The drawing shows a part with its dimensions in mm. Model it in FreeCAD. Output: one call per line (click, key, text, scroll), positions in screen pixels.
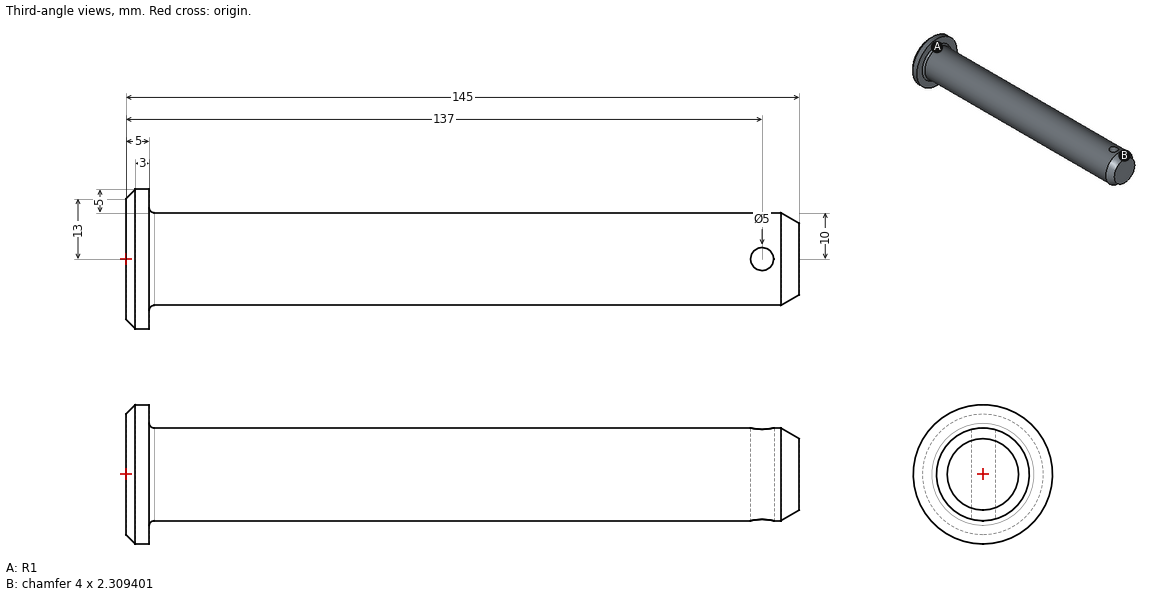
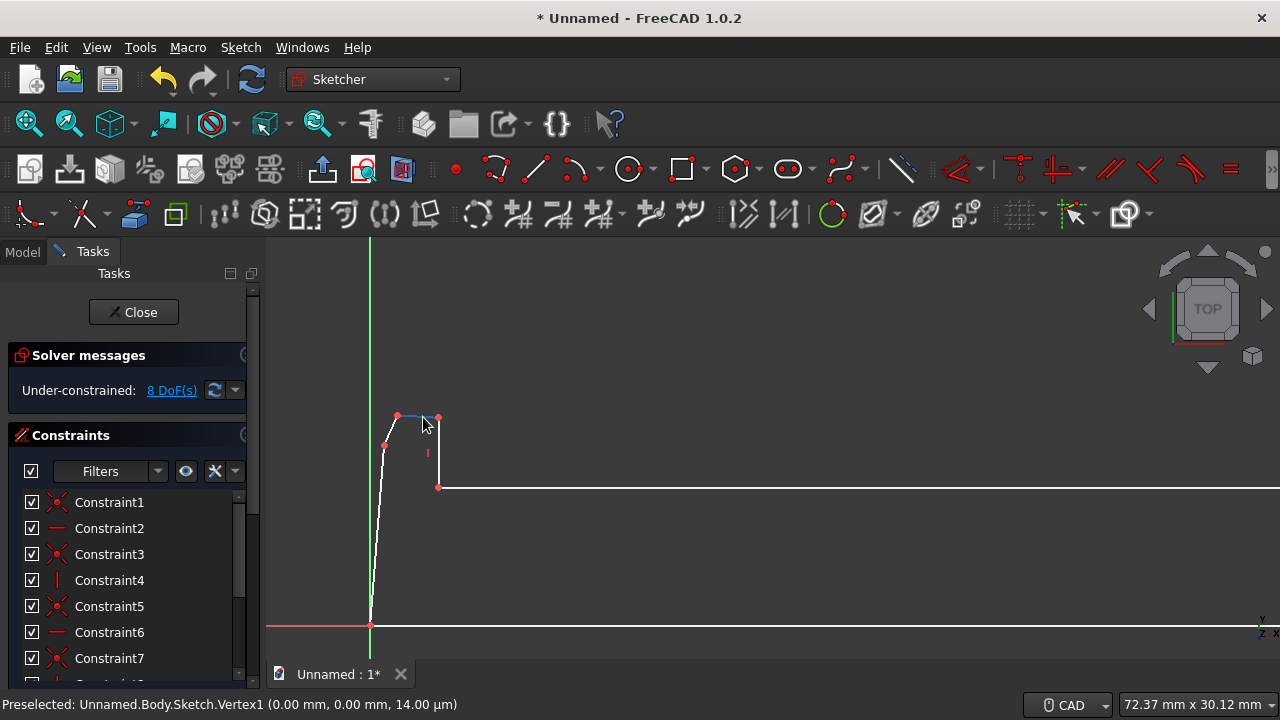
click(422, 417)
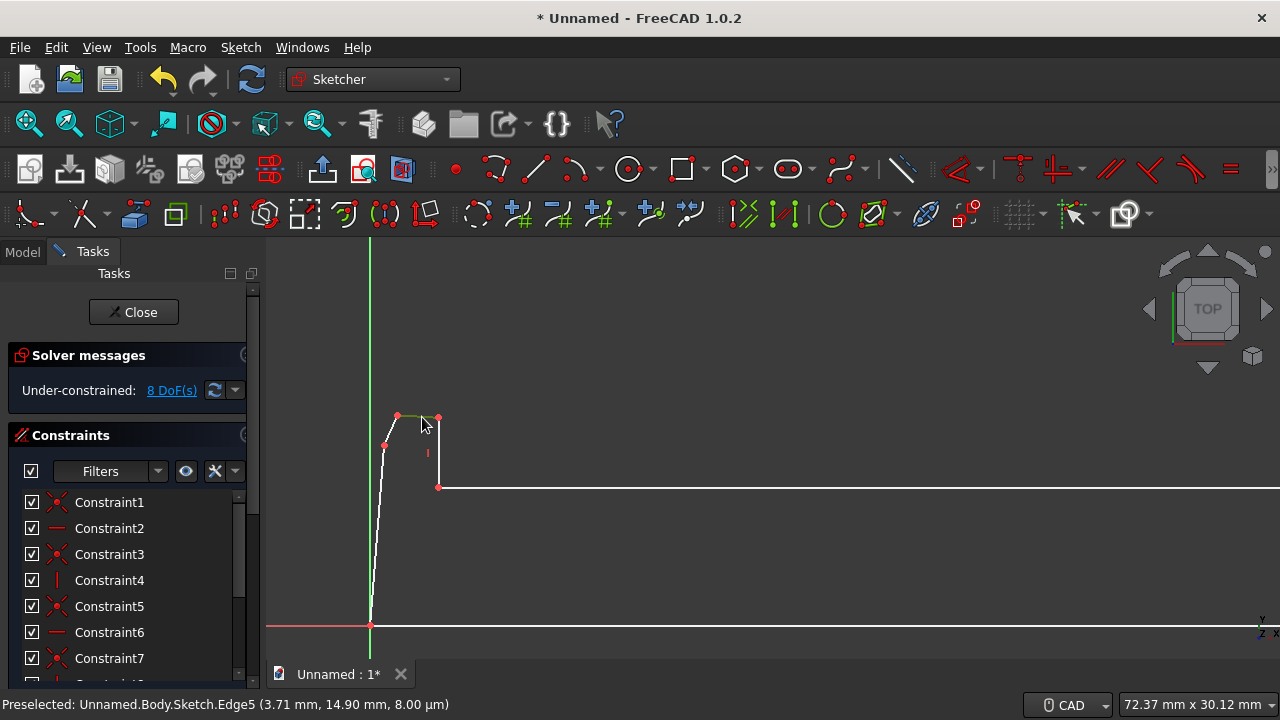
key(h)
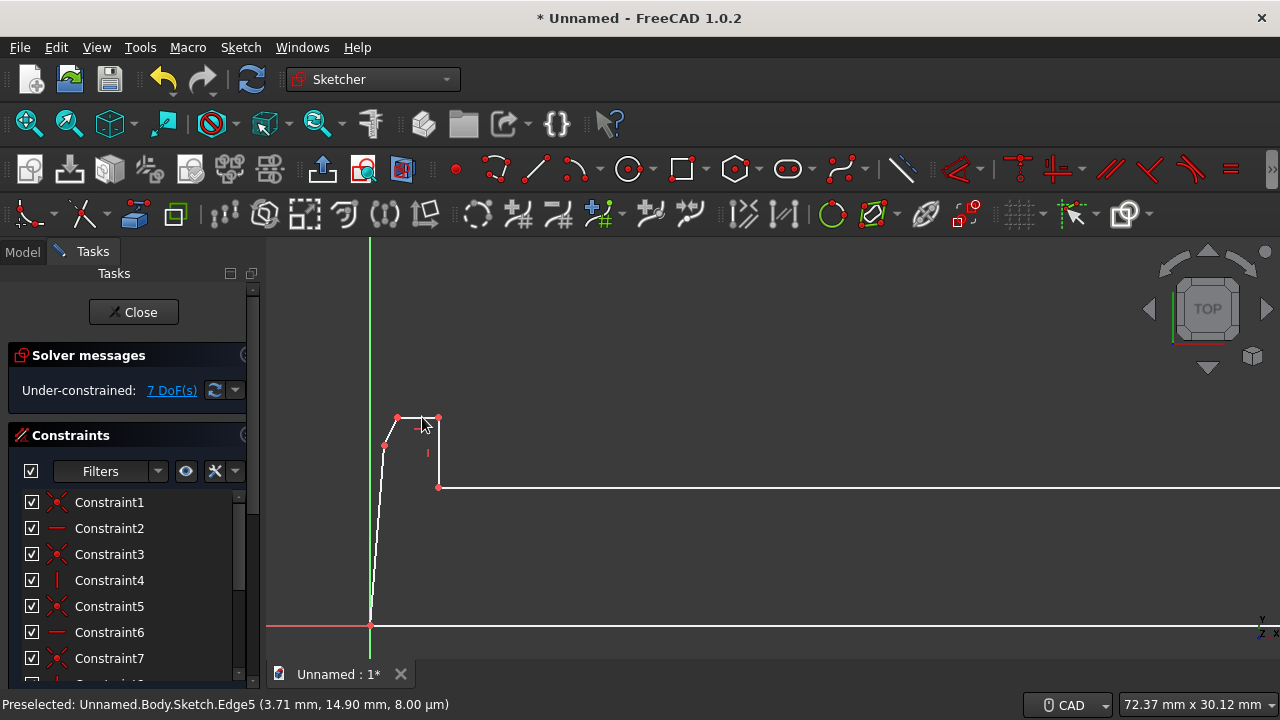
scroll(380, 499, up, 2)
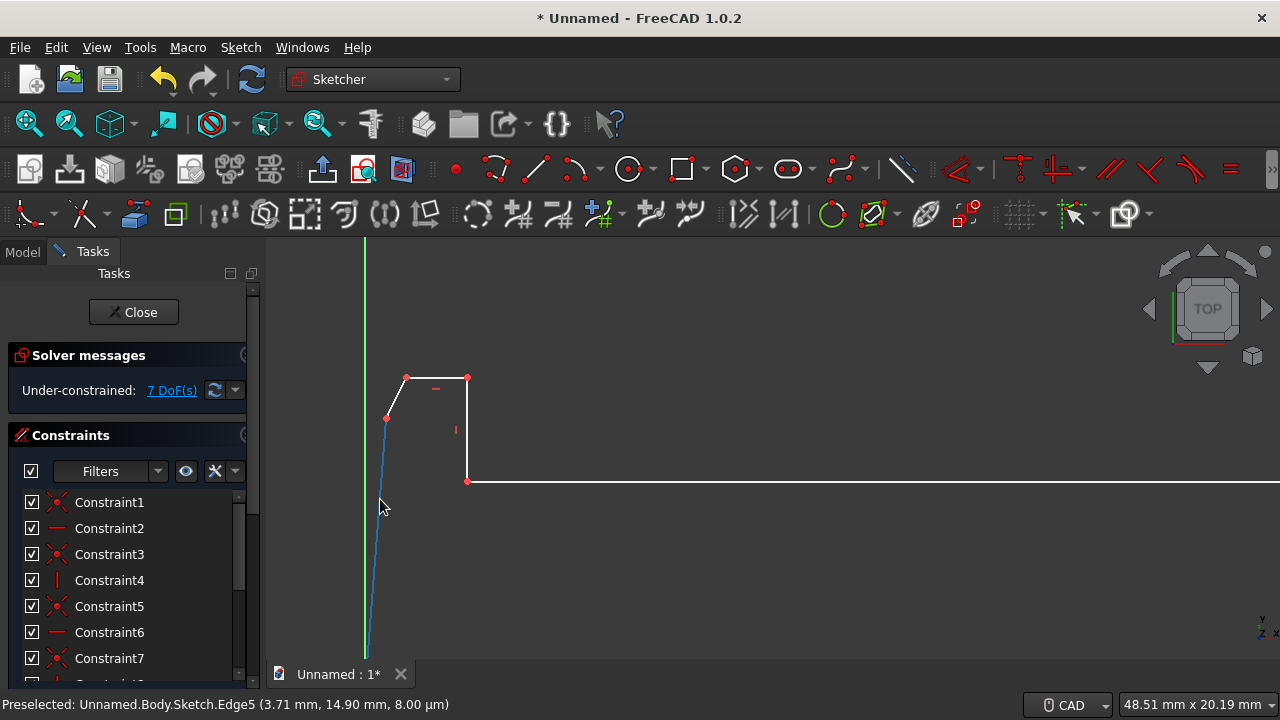
click(380, 499)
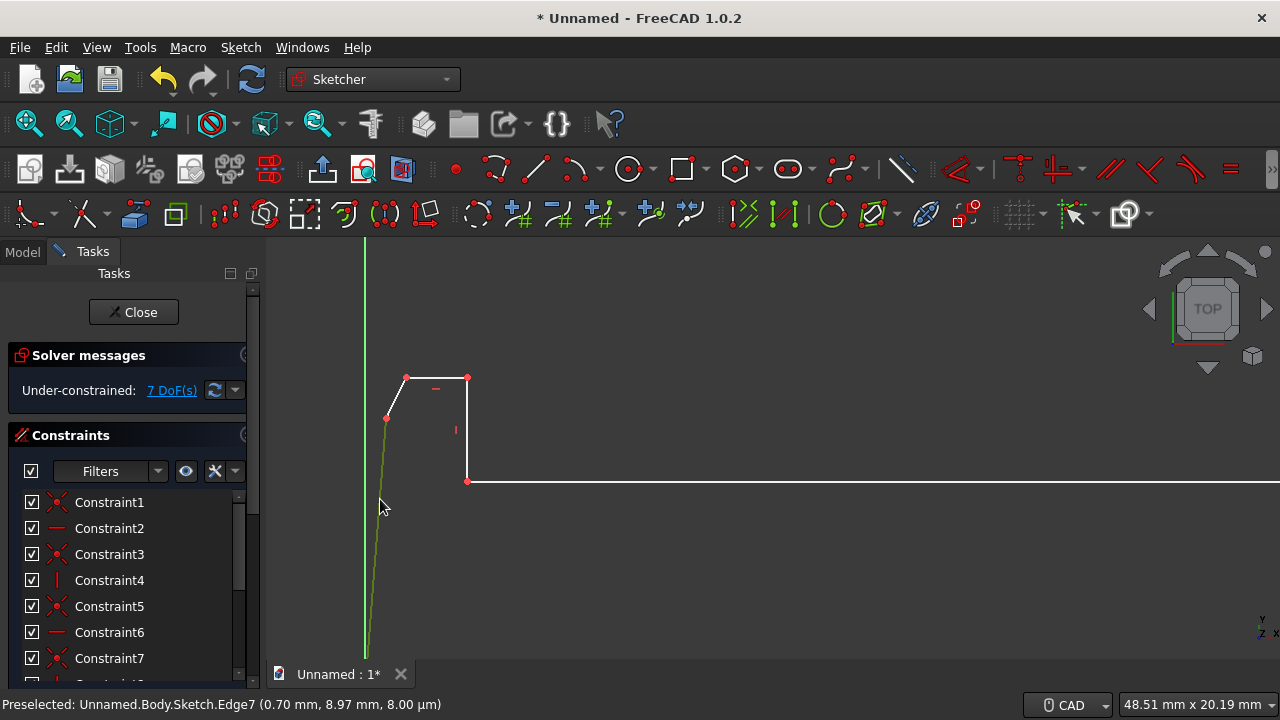
key(v)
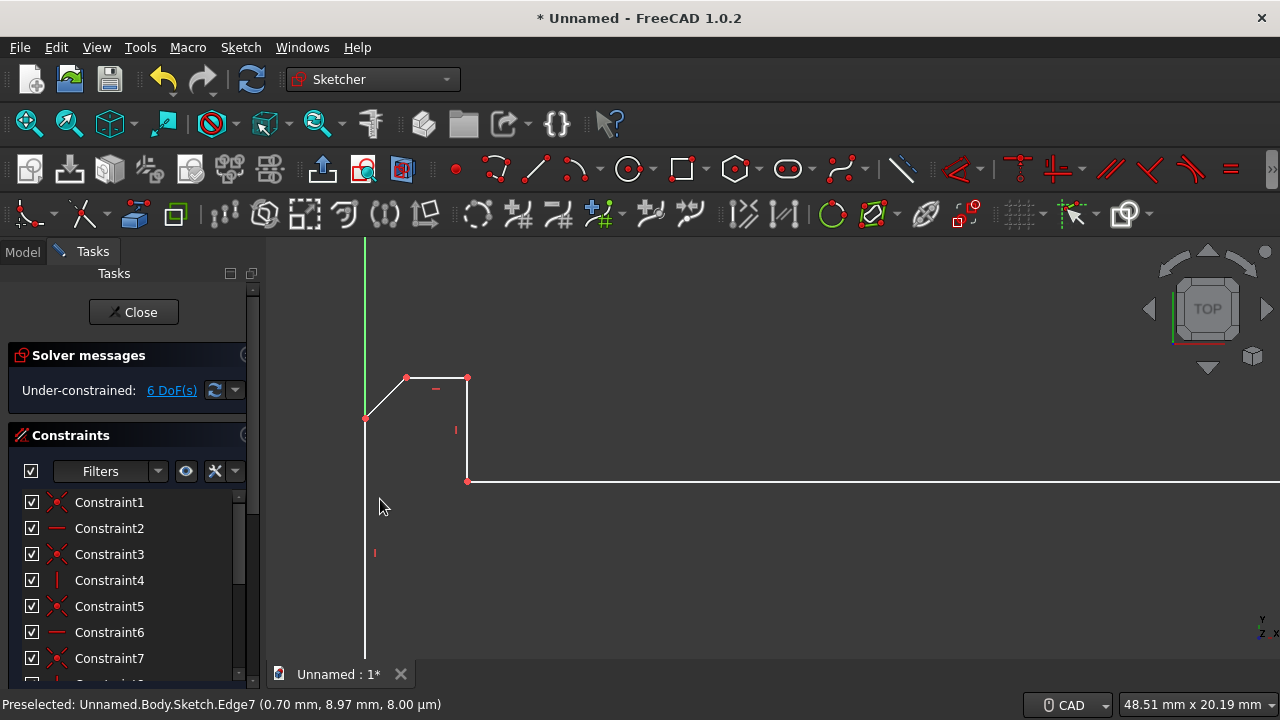
click(467, 450)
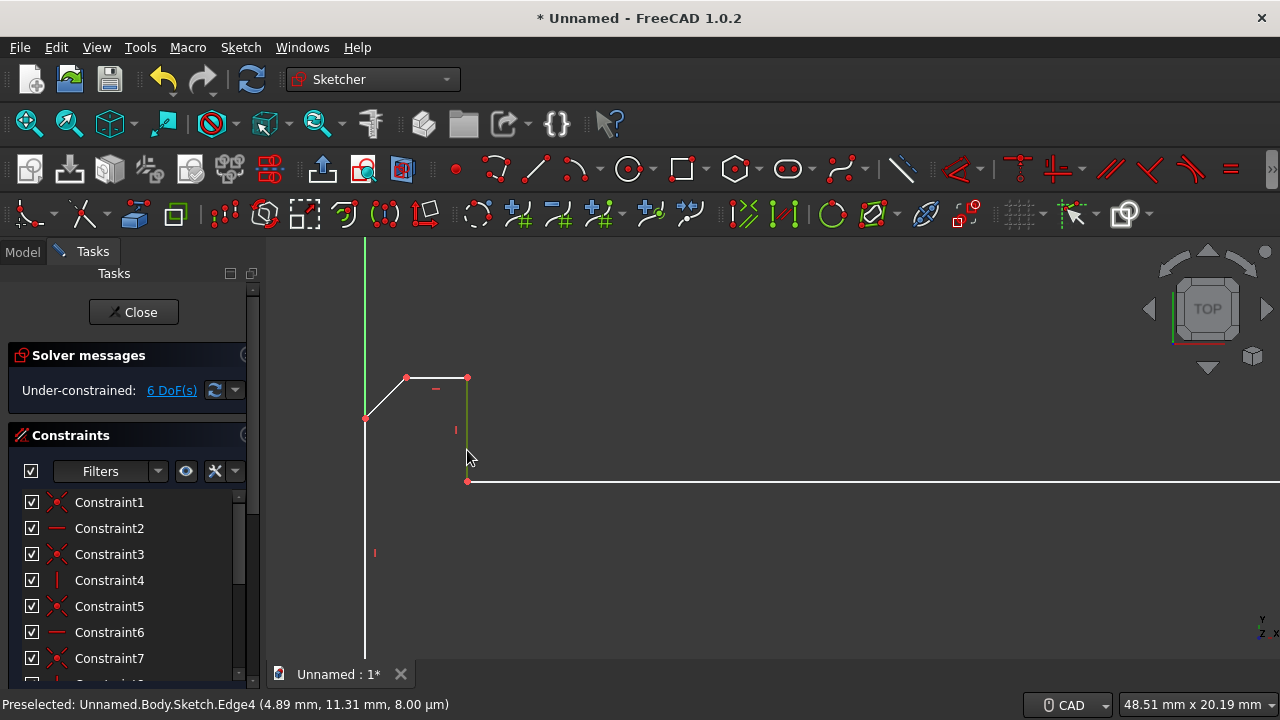
key(i)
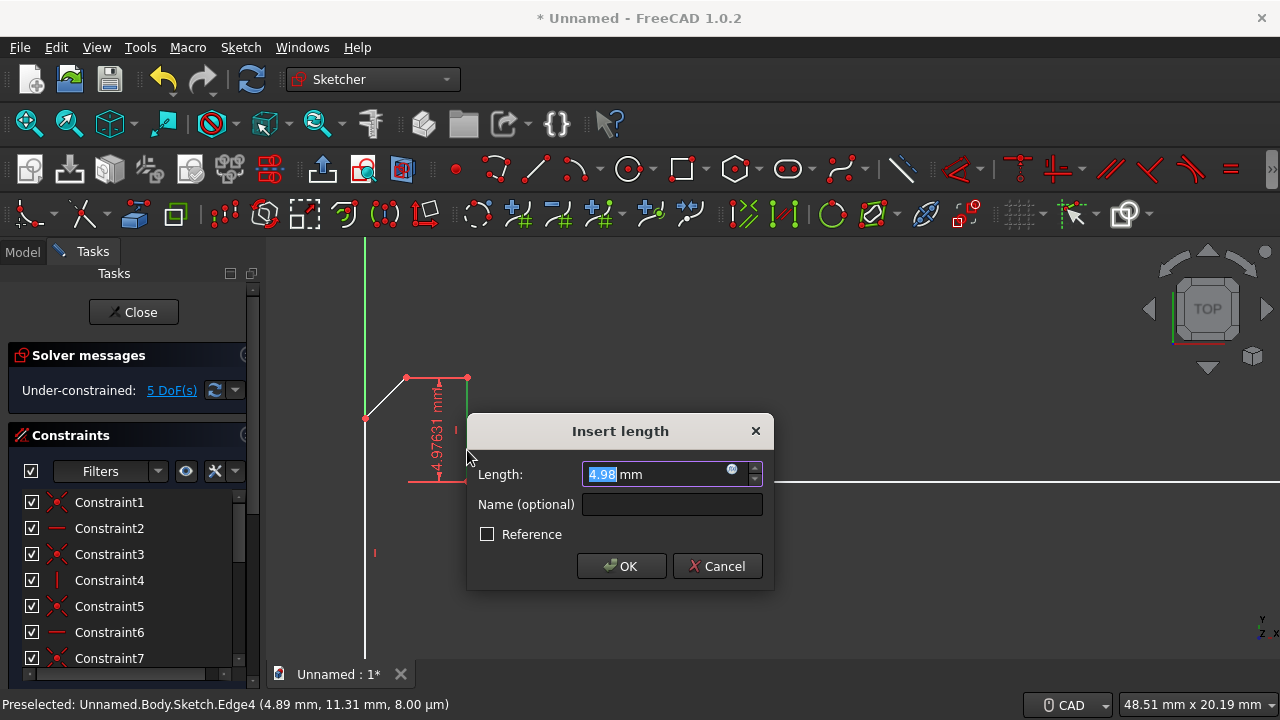
text(5)
key(Return)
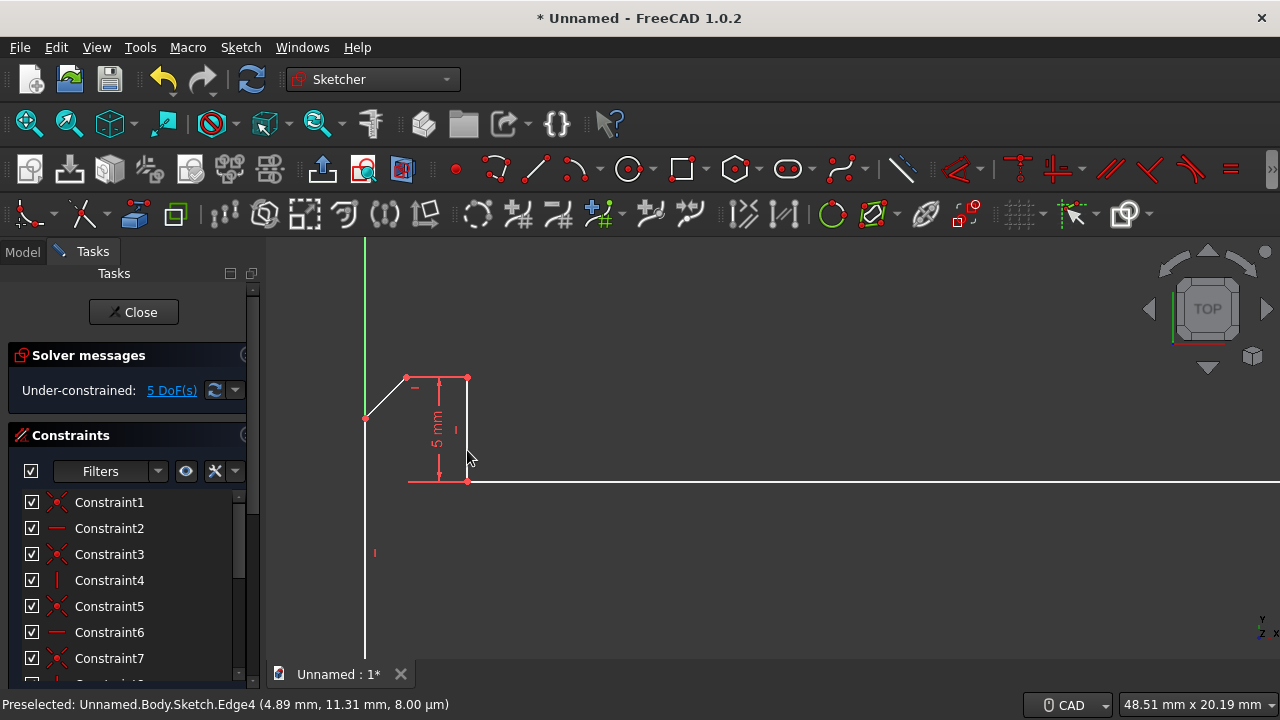
click(449, 377)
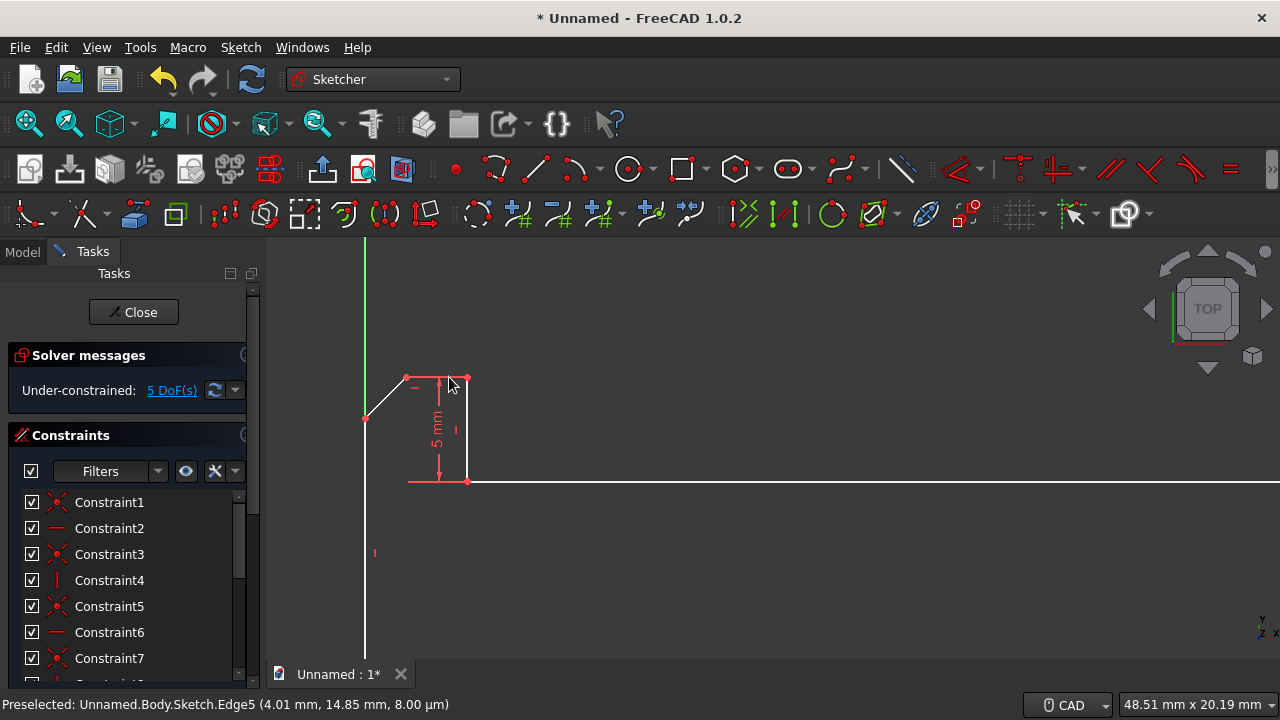
click(982, 170)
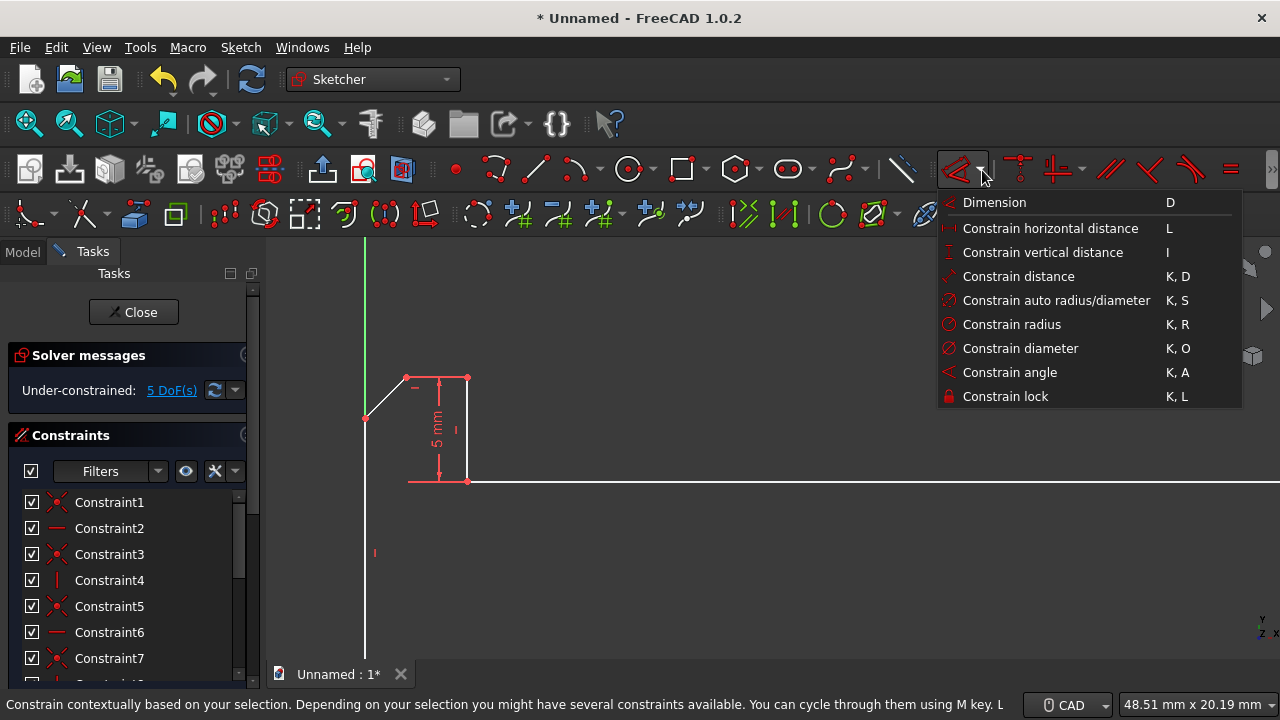
click(1090, 228)